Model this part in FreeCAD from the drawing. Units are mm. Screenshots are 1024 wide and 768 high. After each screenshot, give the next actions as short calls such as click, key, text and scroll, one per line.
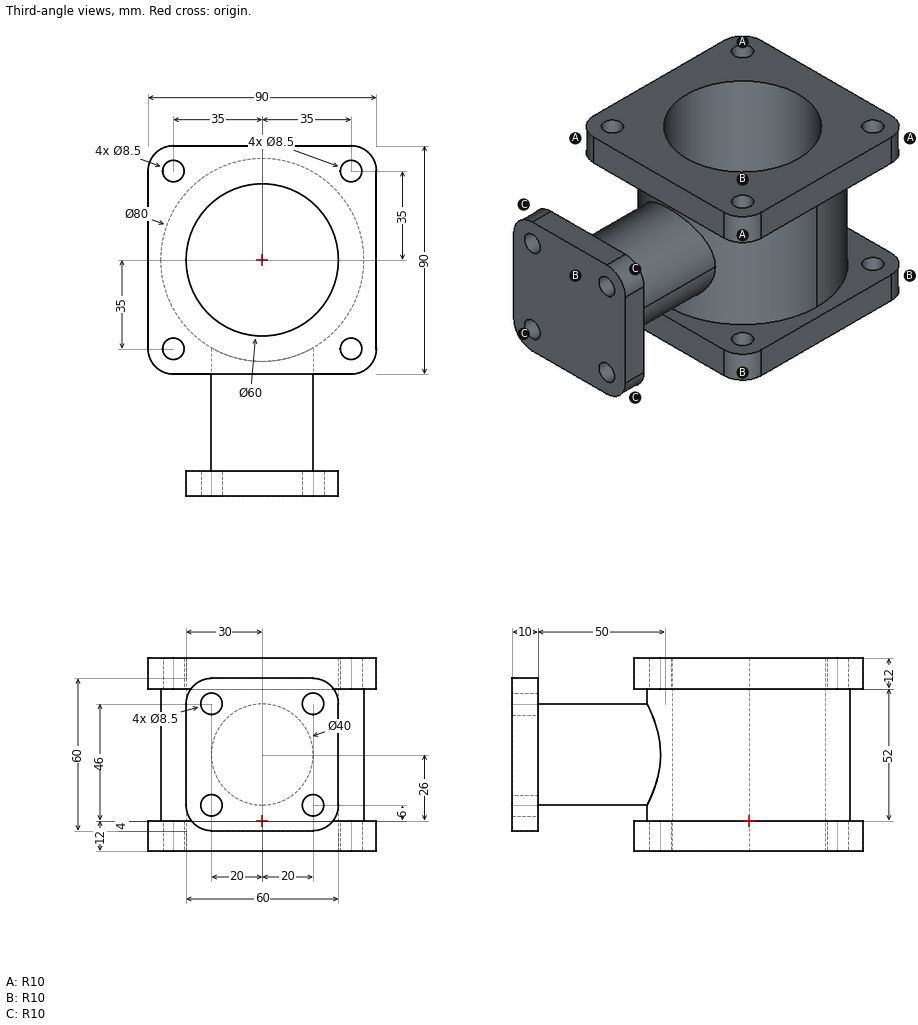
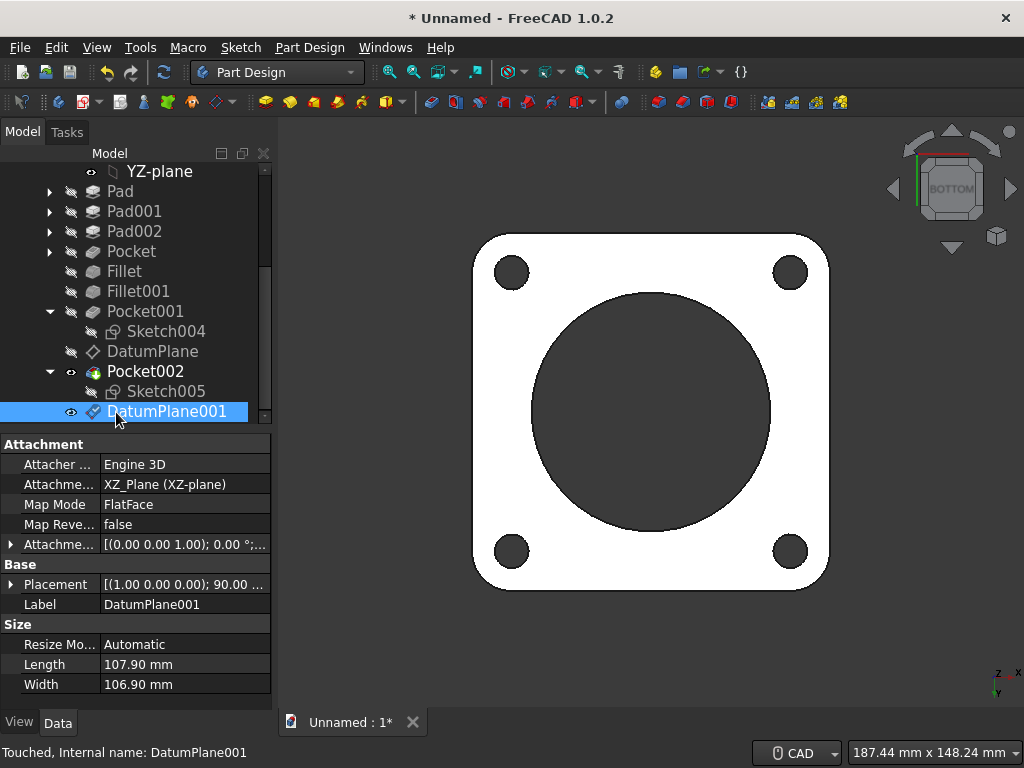
click(84, 102)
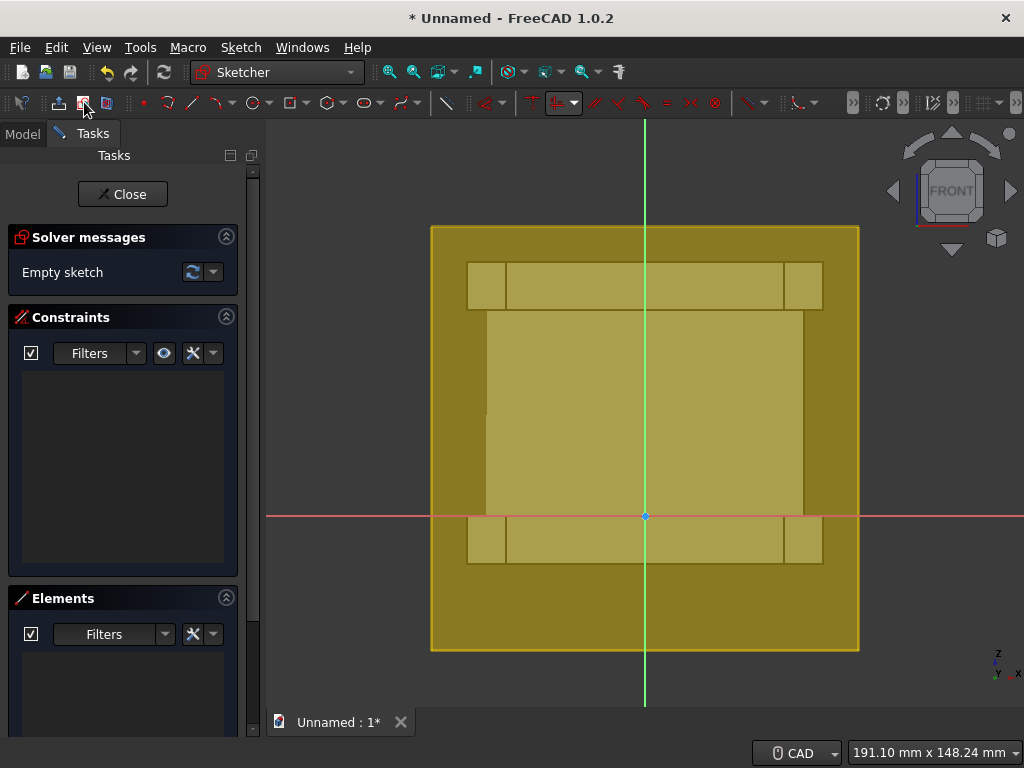
scroll(701, 435, up, 4)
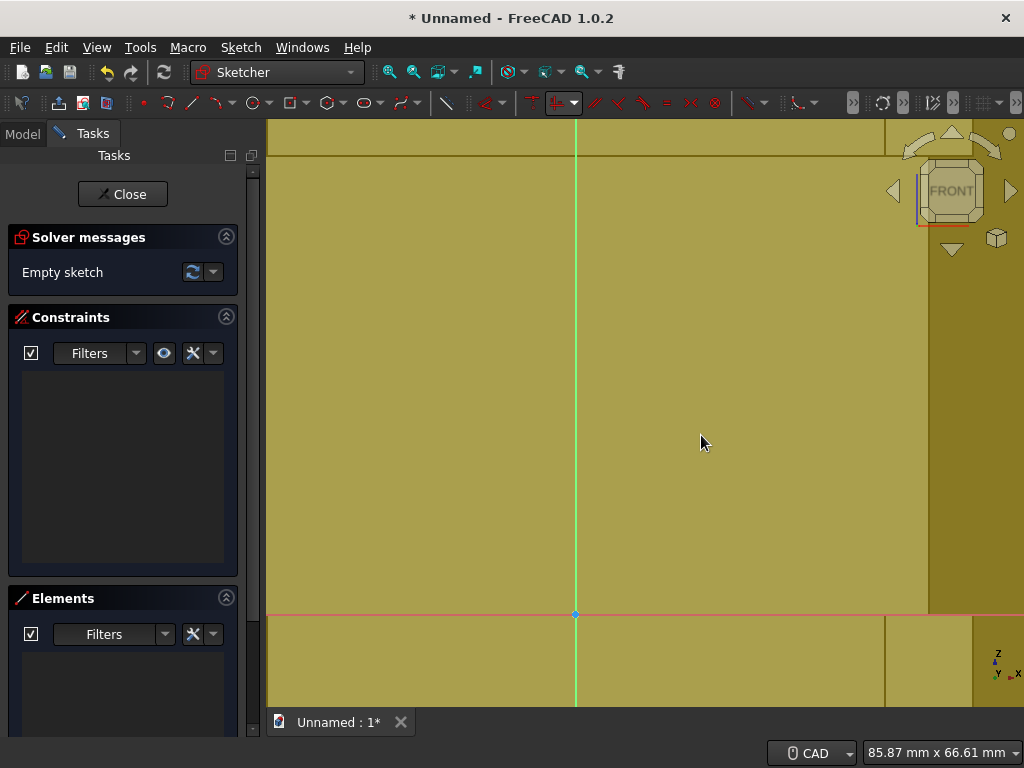
click(254, 104)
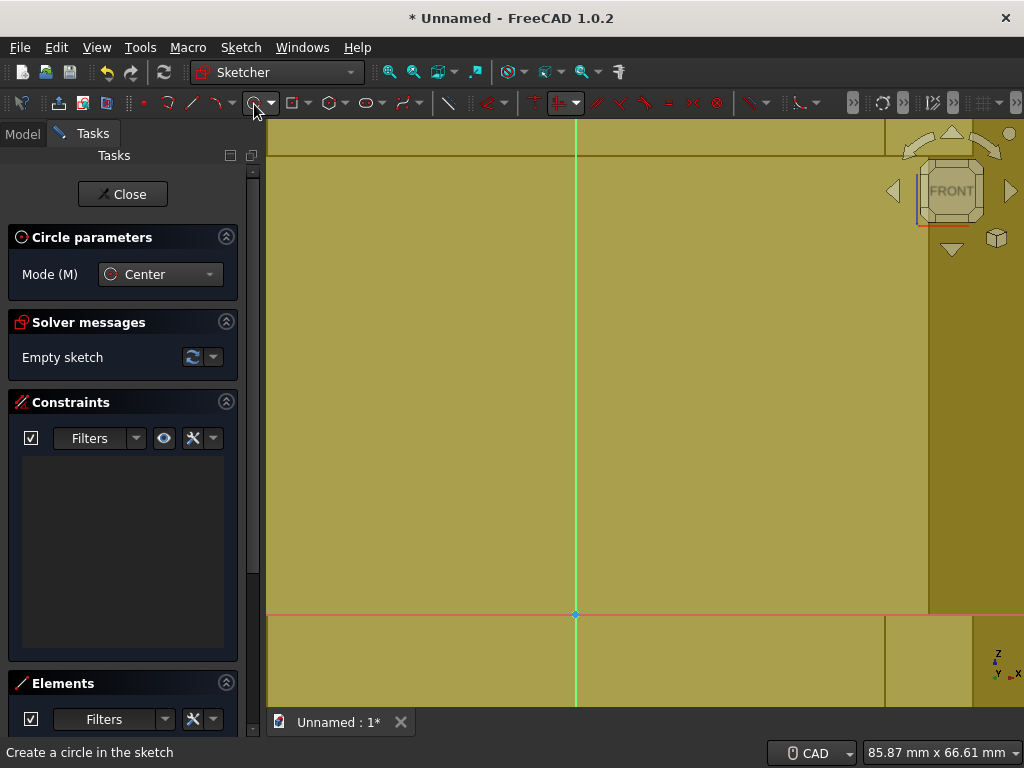
click(576, 385)
click(701, 261)
key(Escape)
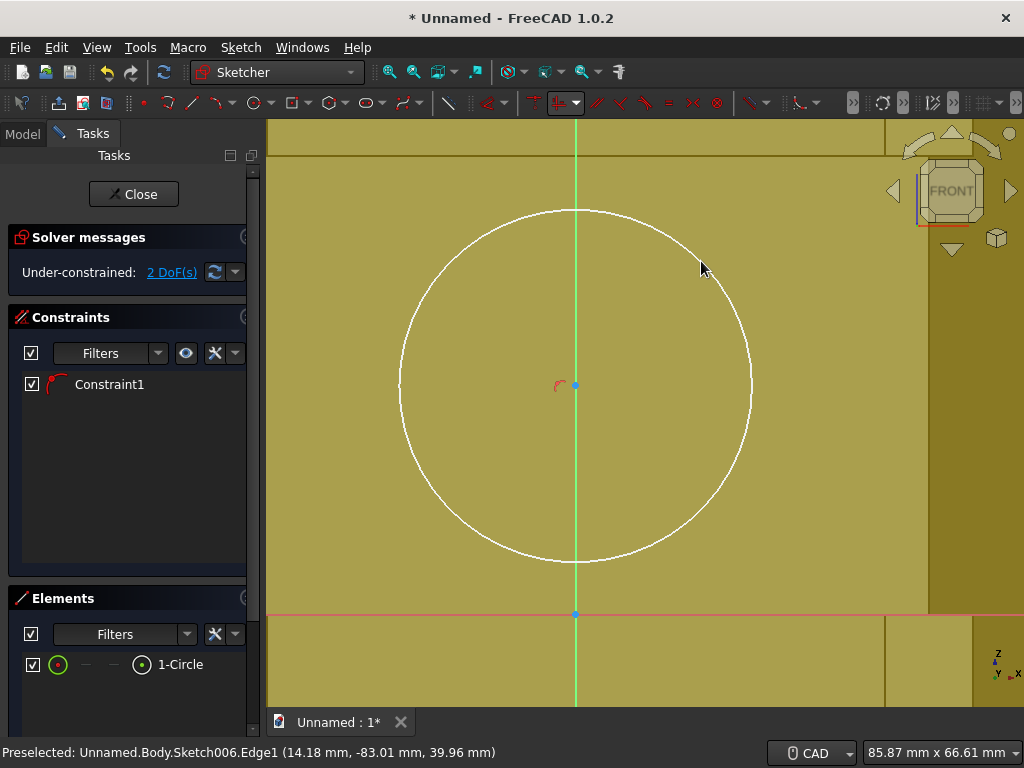
key(d)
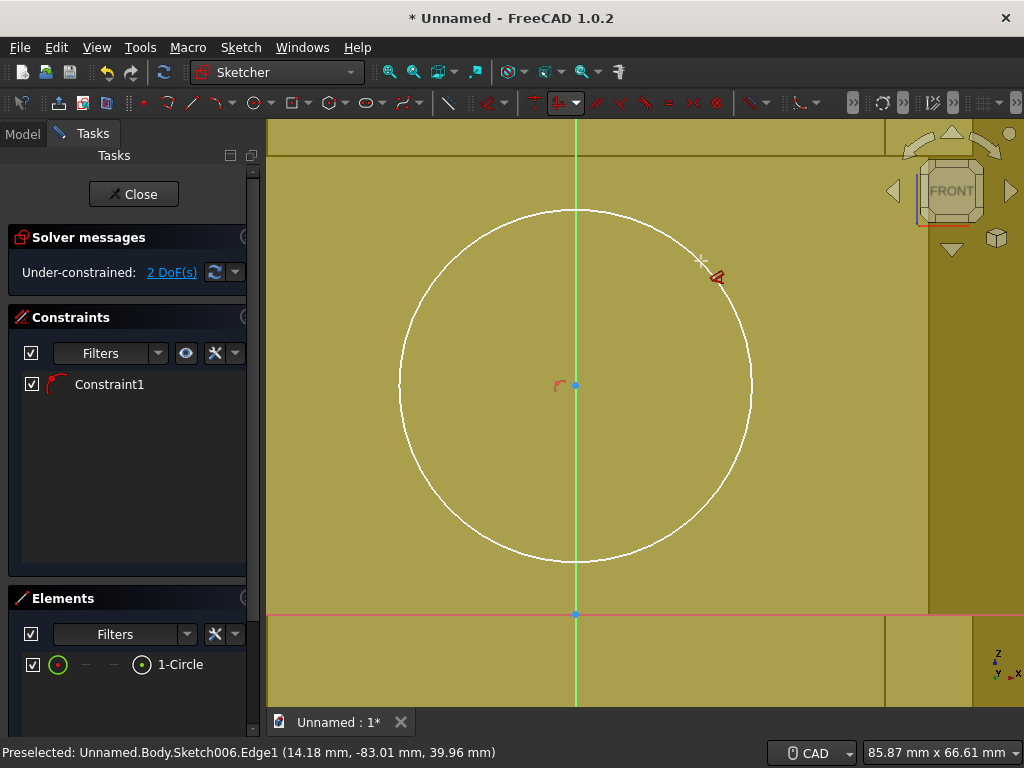
click(700, 261)
click(723, 238)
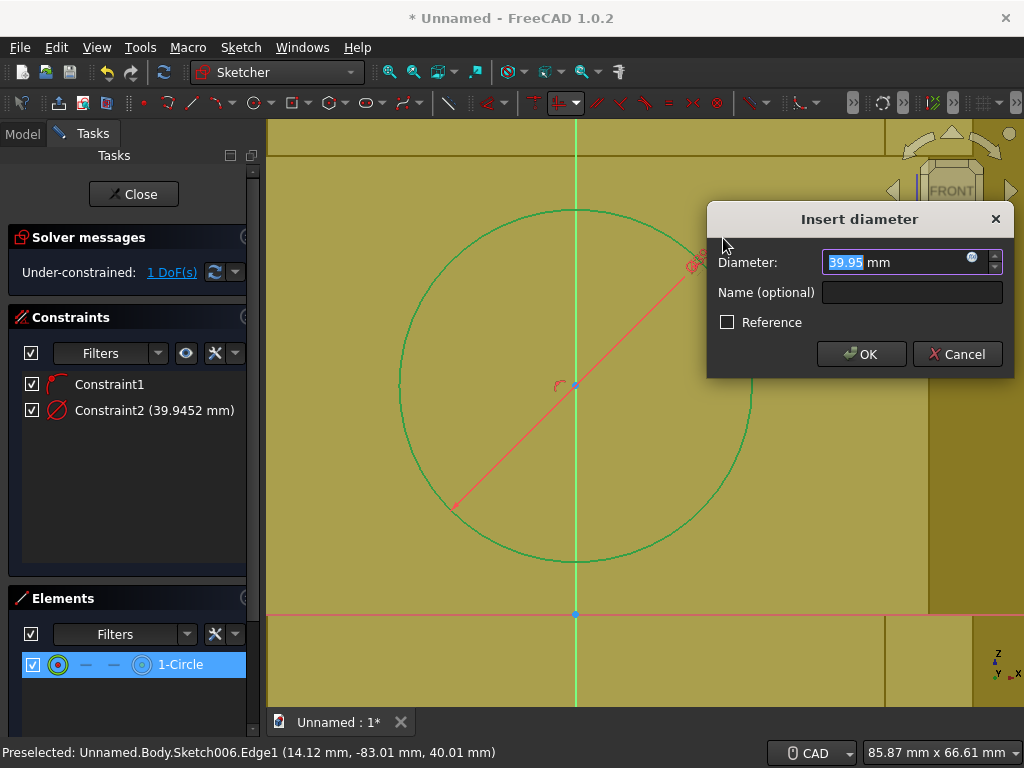
text(40)
key(Return)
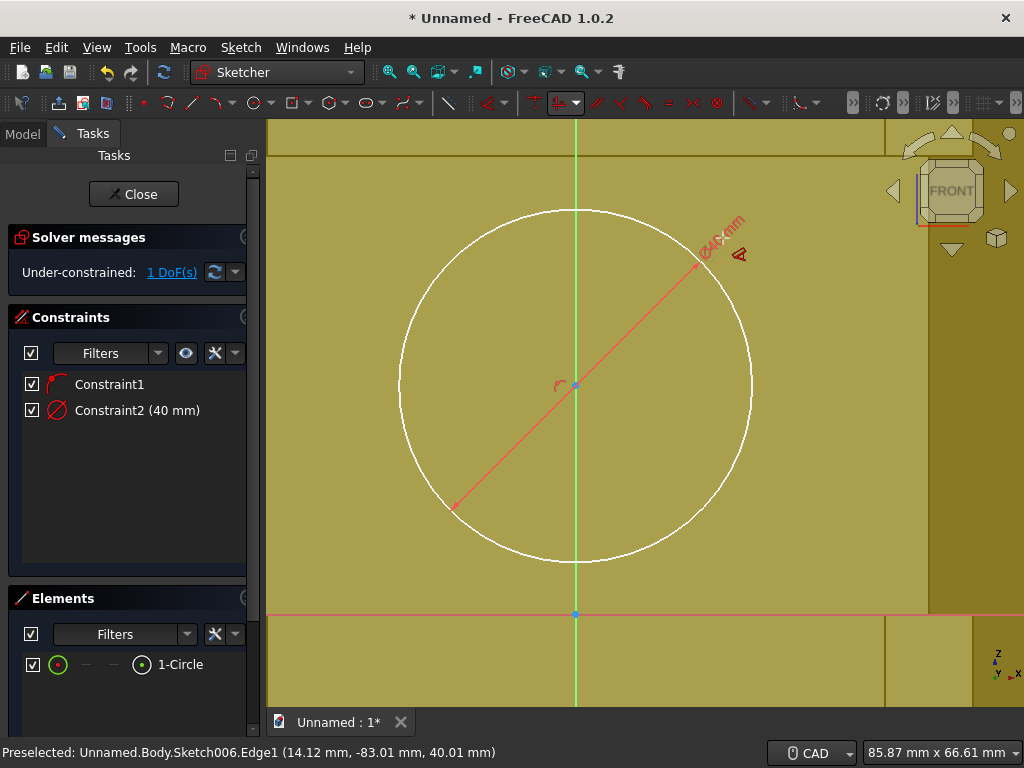
click(576, 386)
click(610, 500)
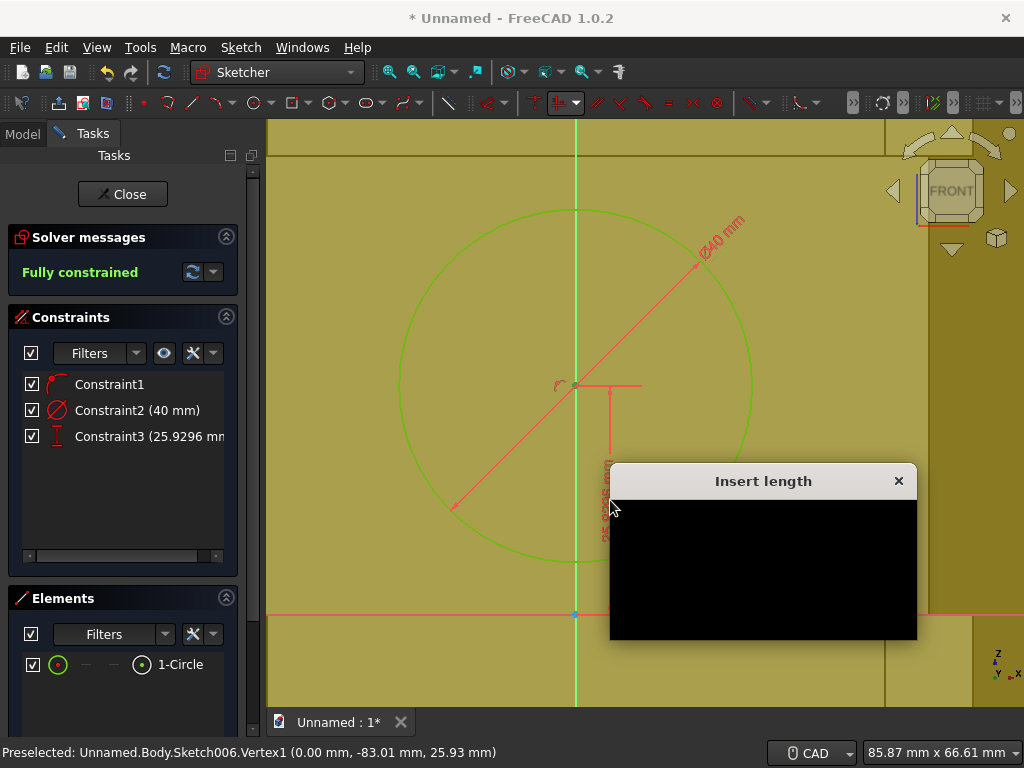
text(26)
key(Return)
key(Escape)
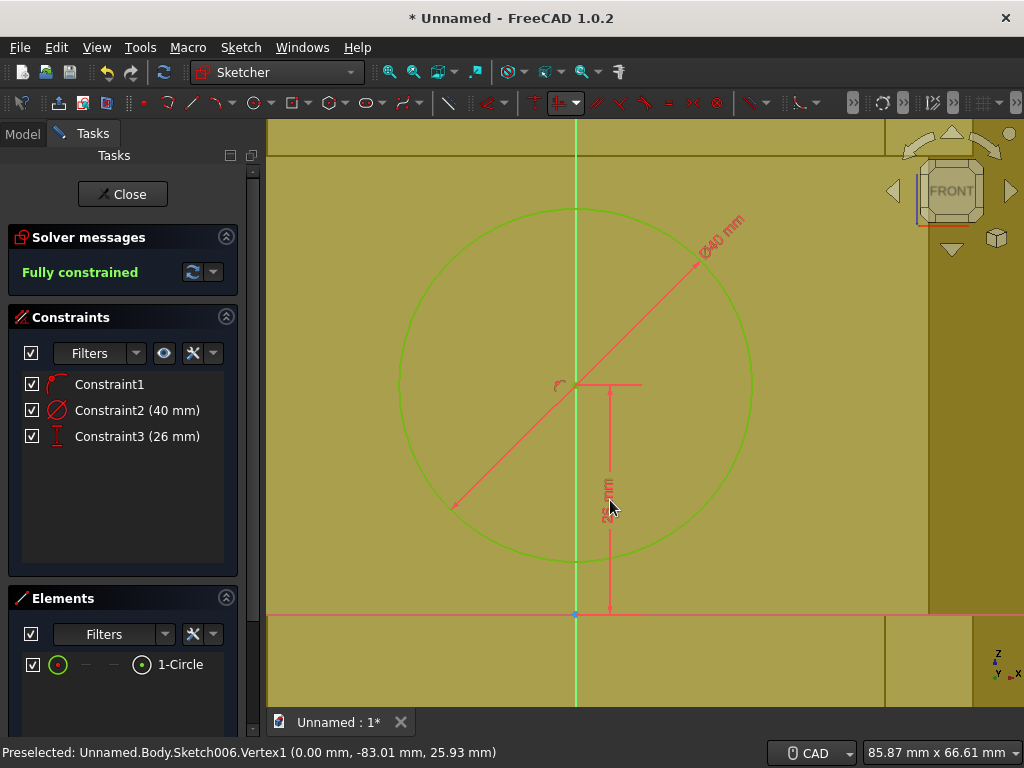
click(123, 194)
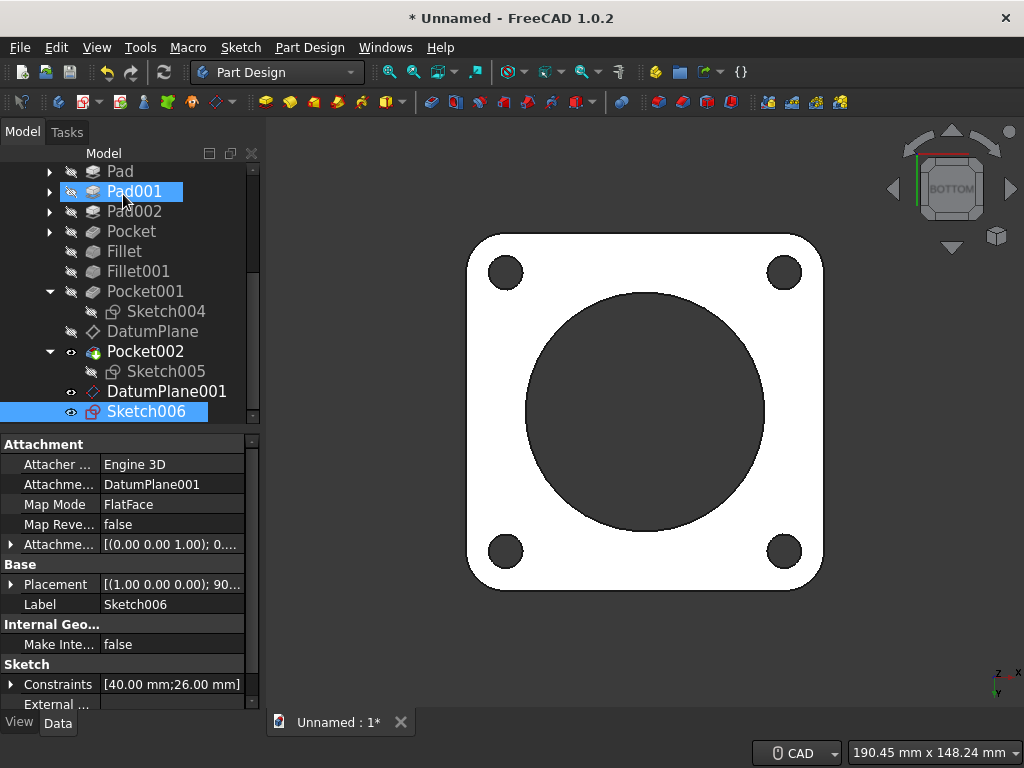
click(266, 102)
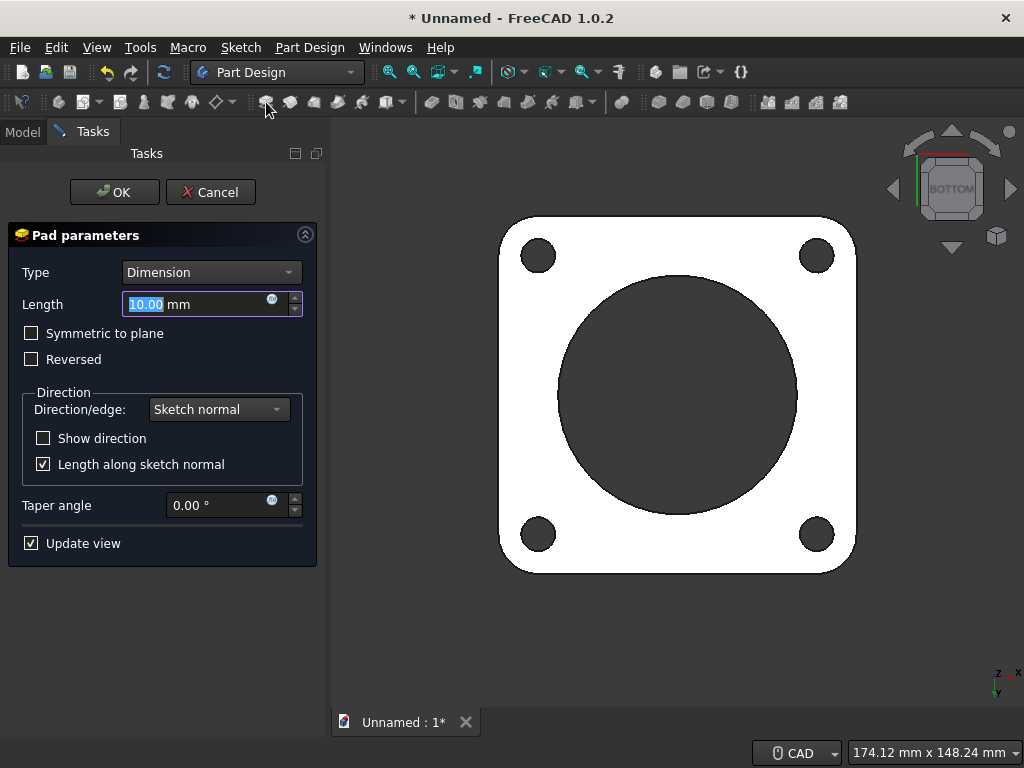
text(50)
key(Tab)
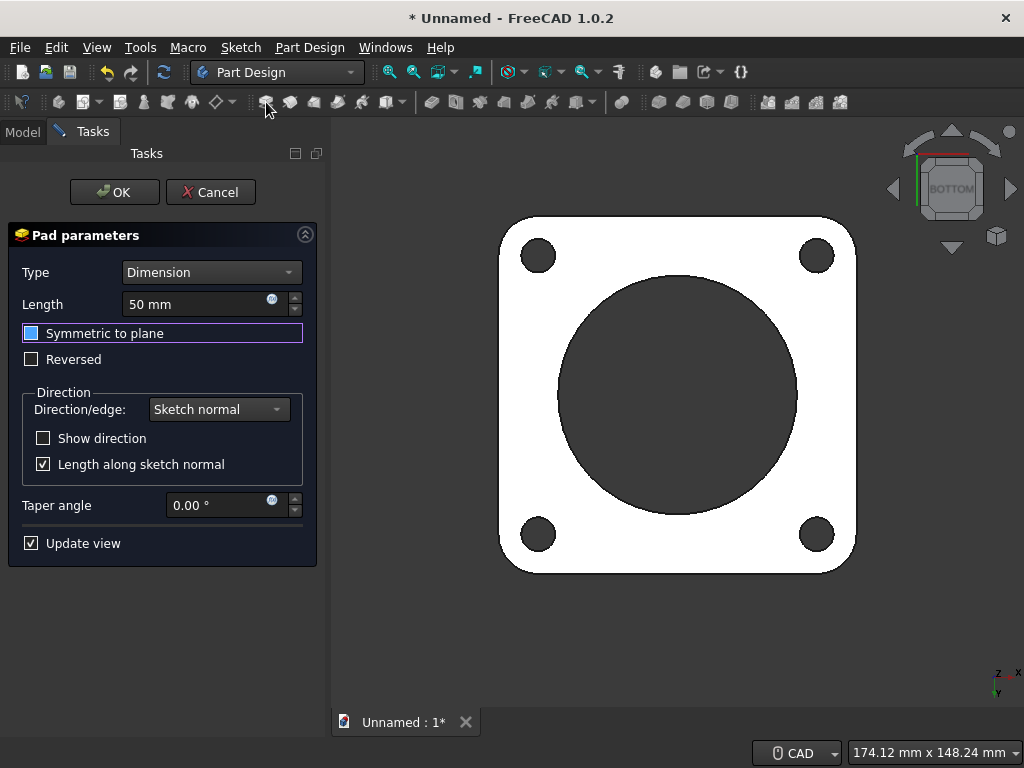
click(30, 359)